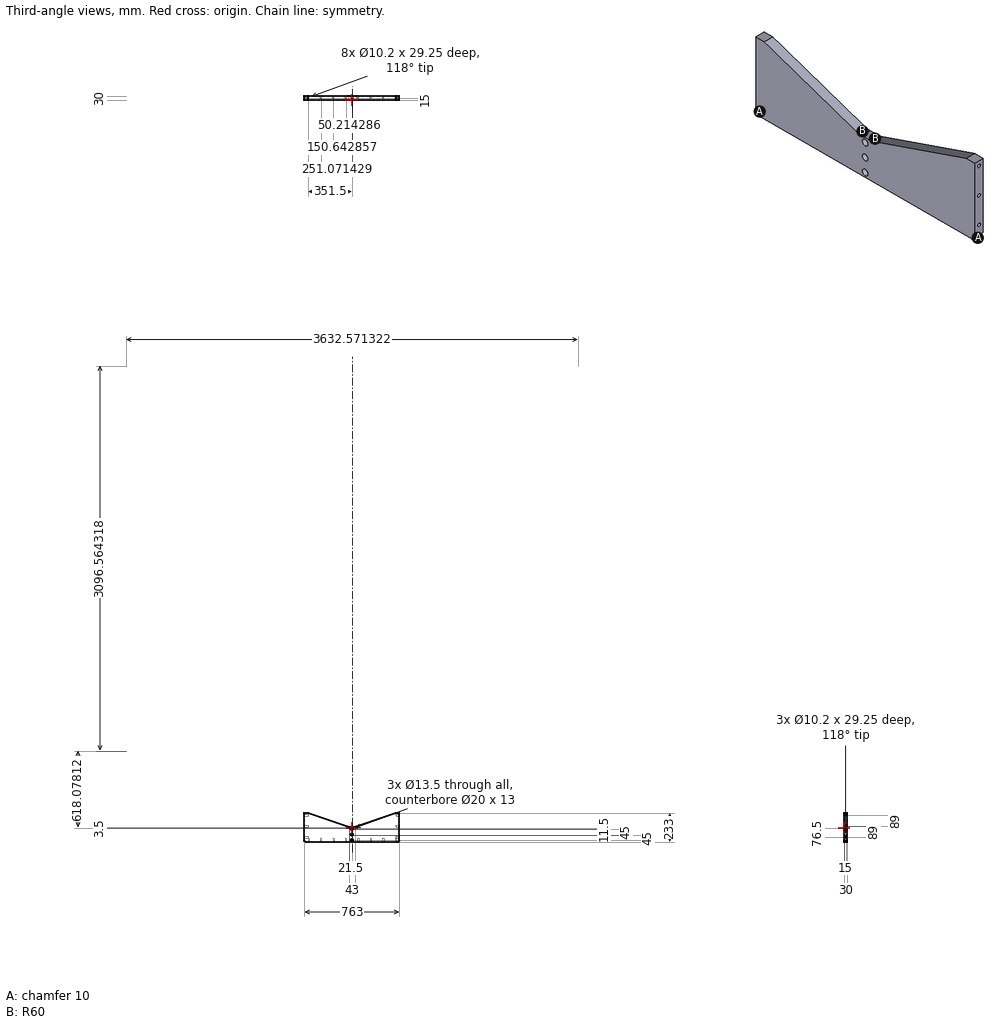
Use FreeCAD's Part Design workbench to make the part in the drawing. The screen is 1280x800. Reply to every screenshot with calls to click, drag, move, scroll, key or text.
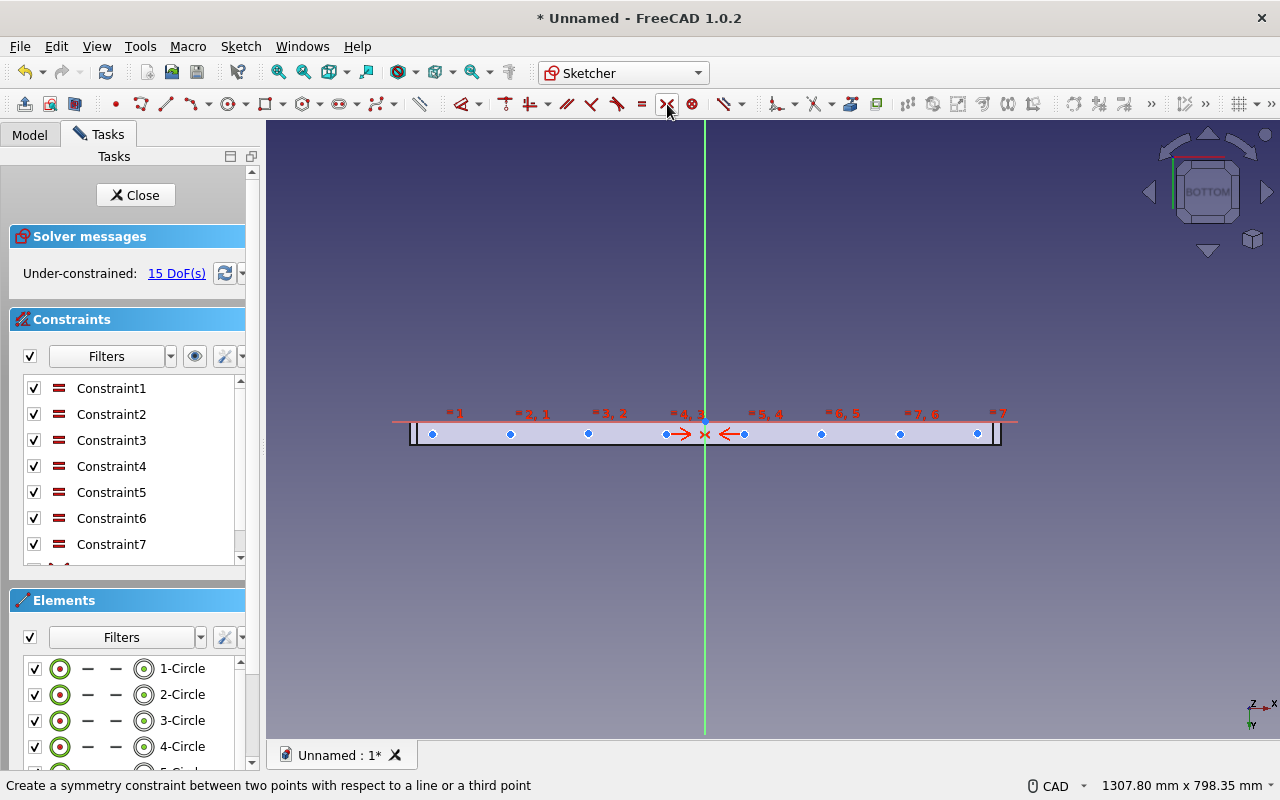
click(588, 434)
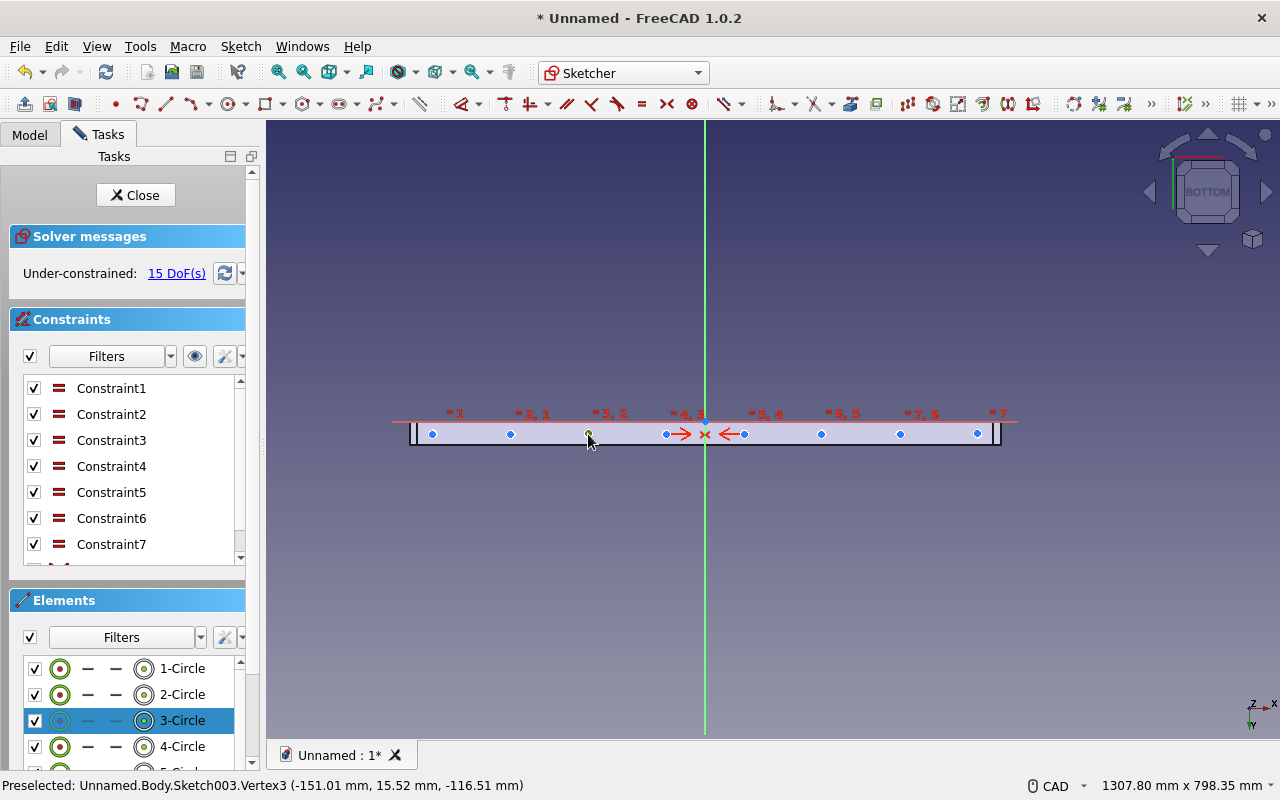
click(822, 434)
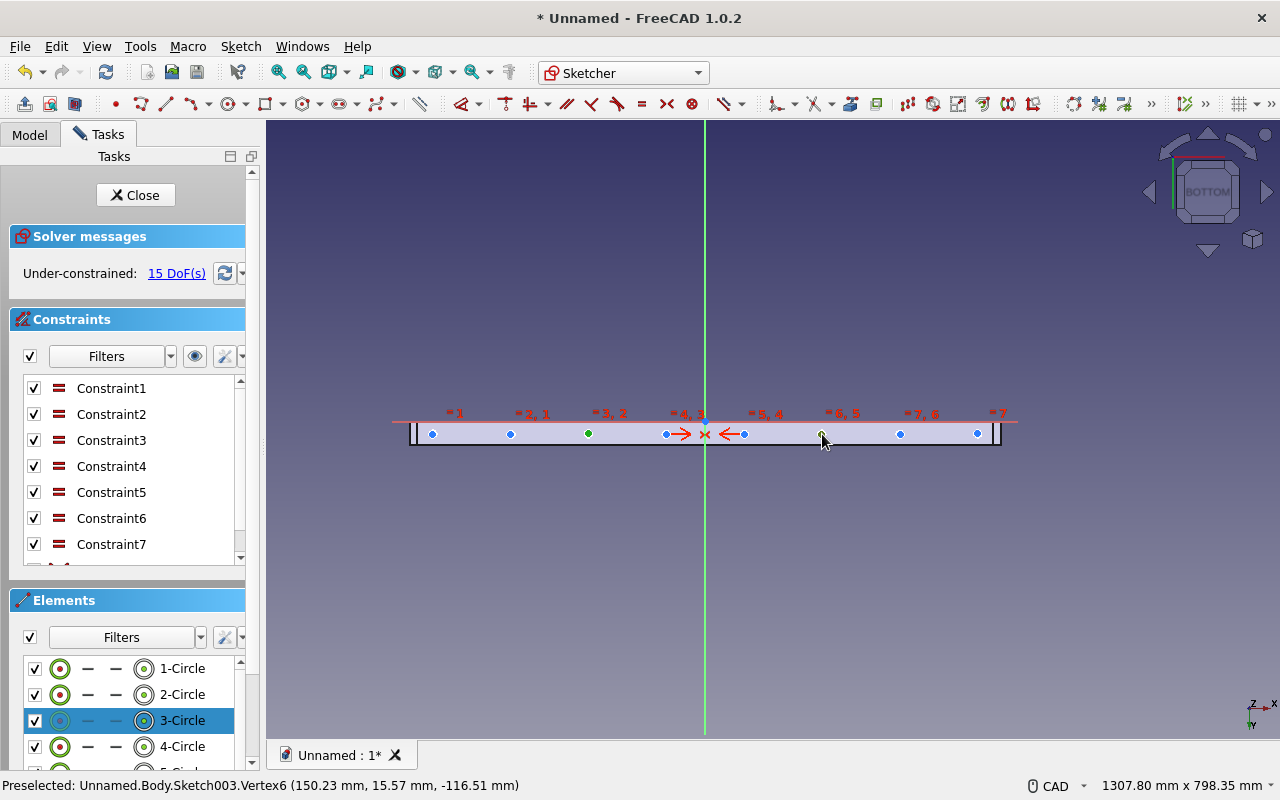
click(705, 671)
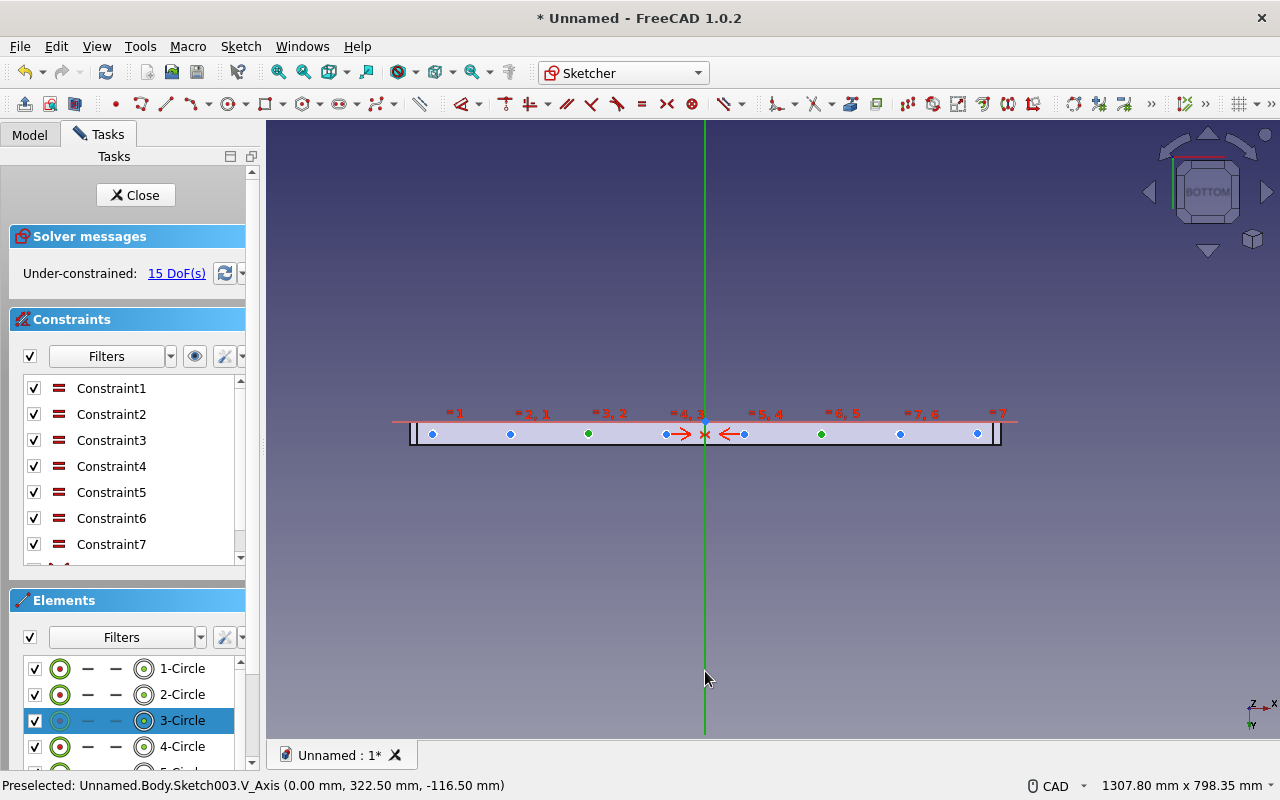
key(s)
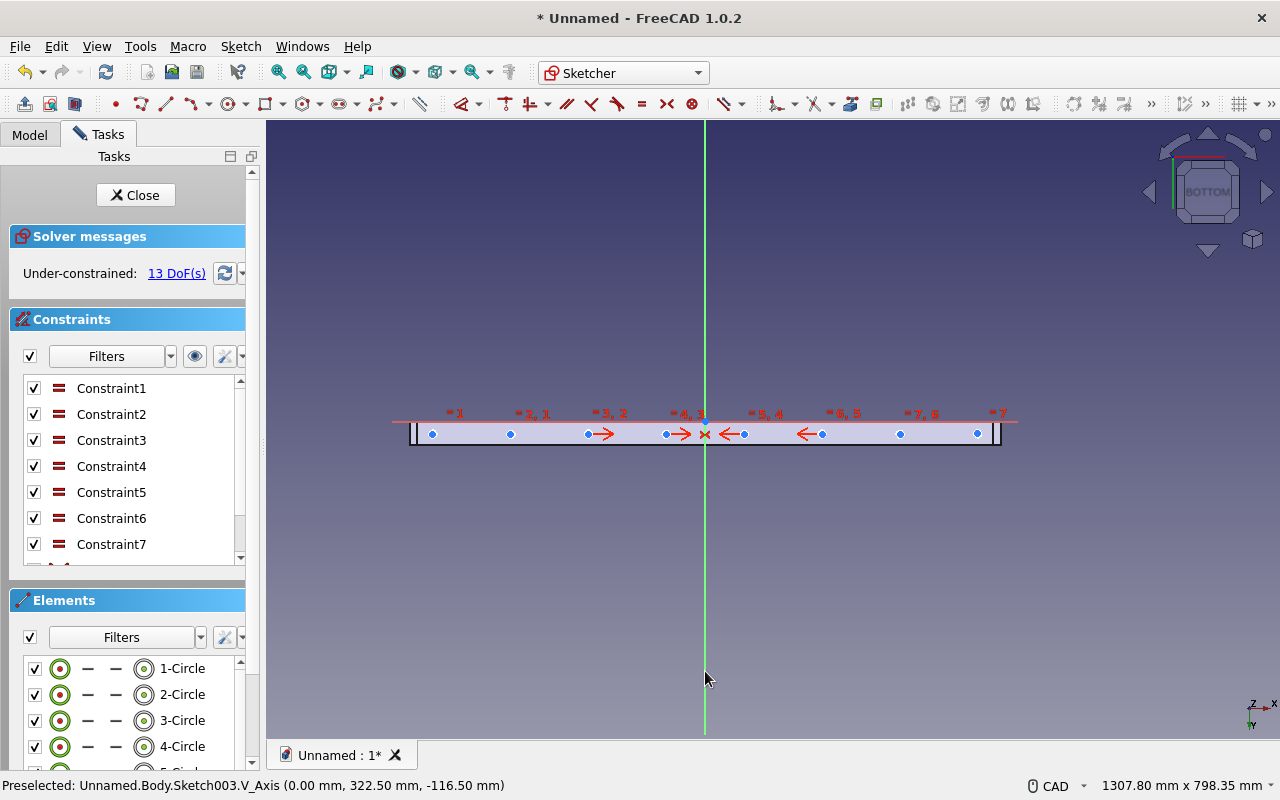
click(511, 435)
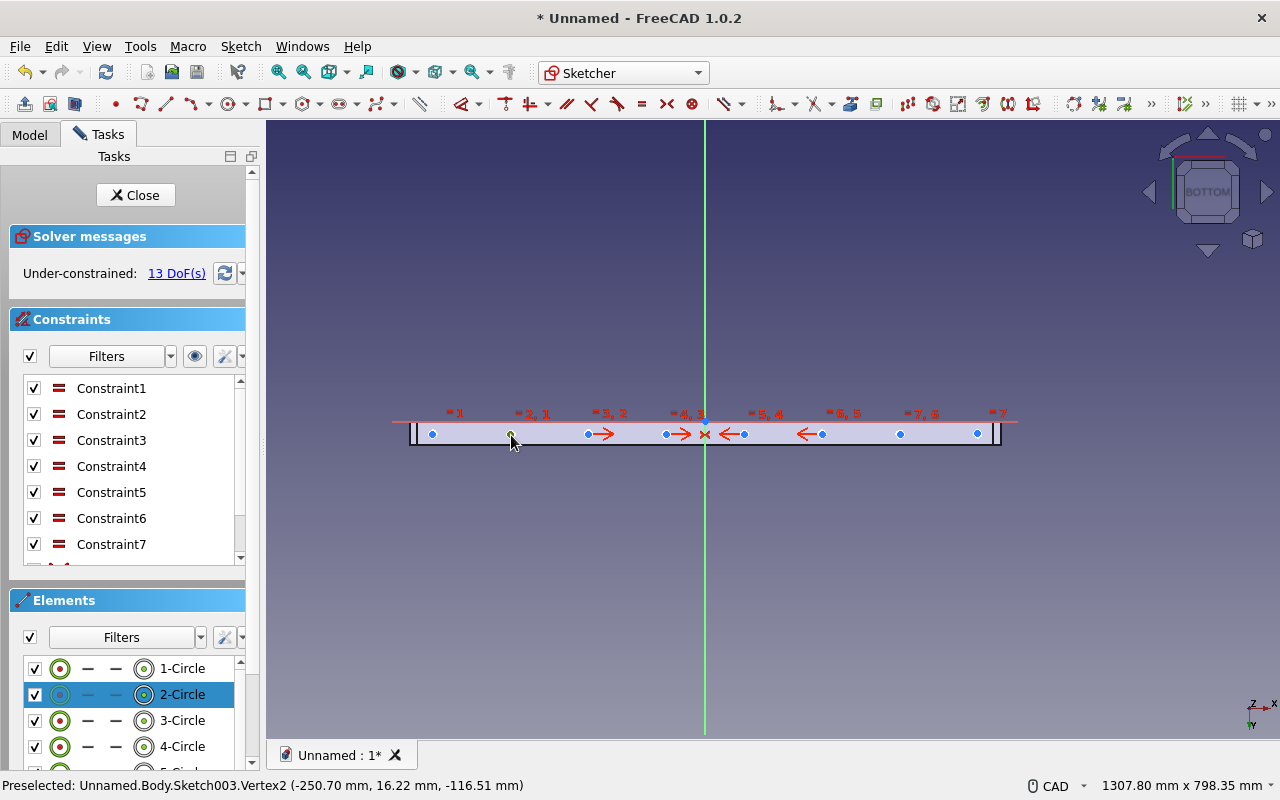
click(900, 434)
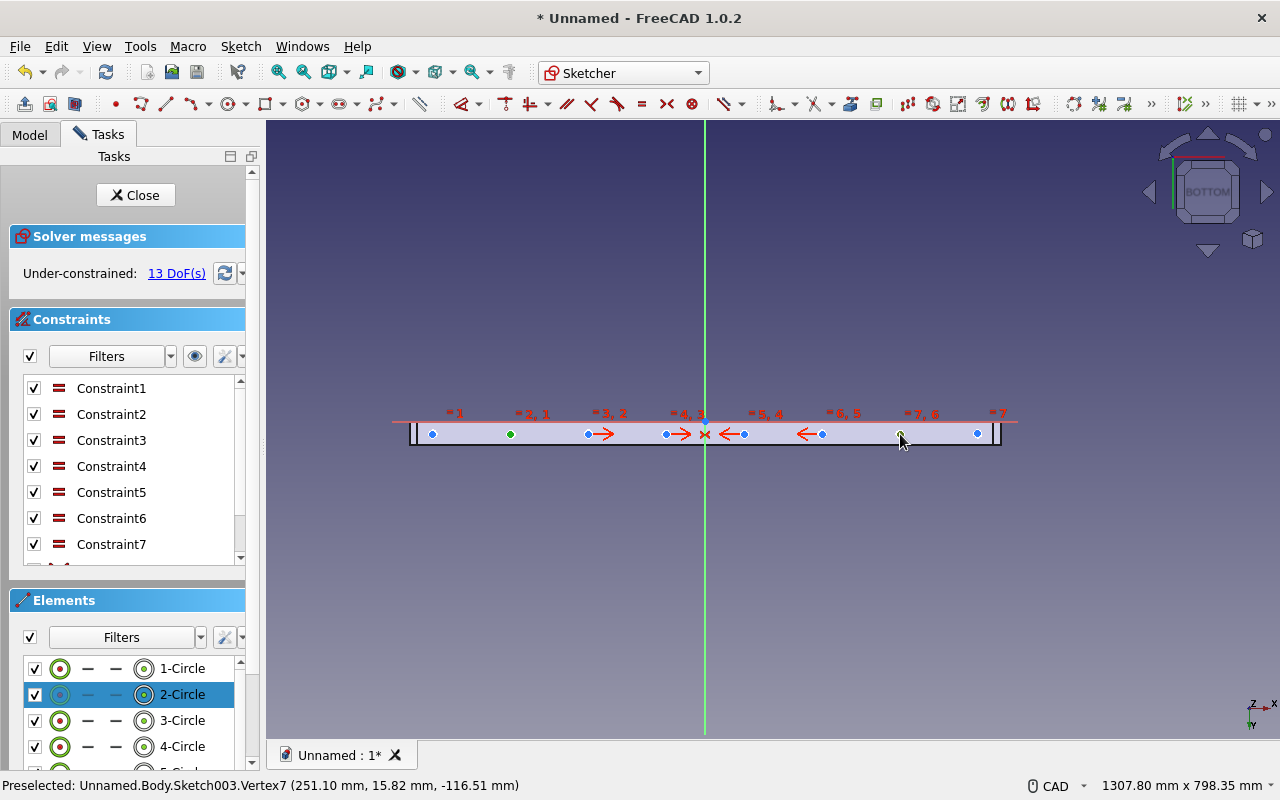
click(705, 671)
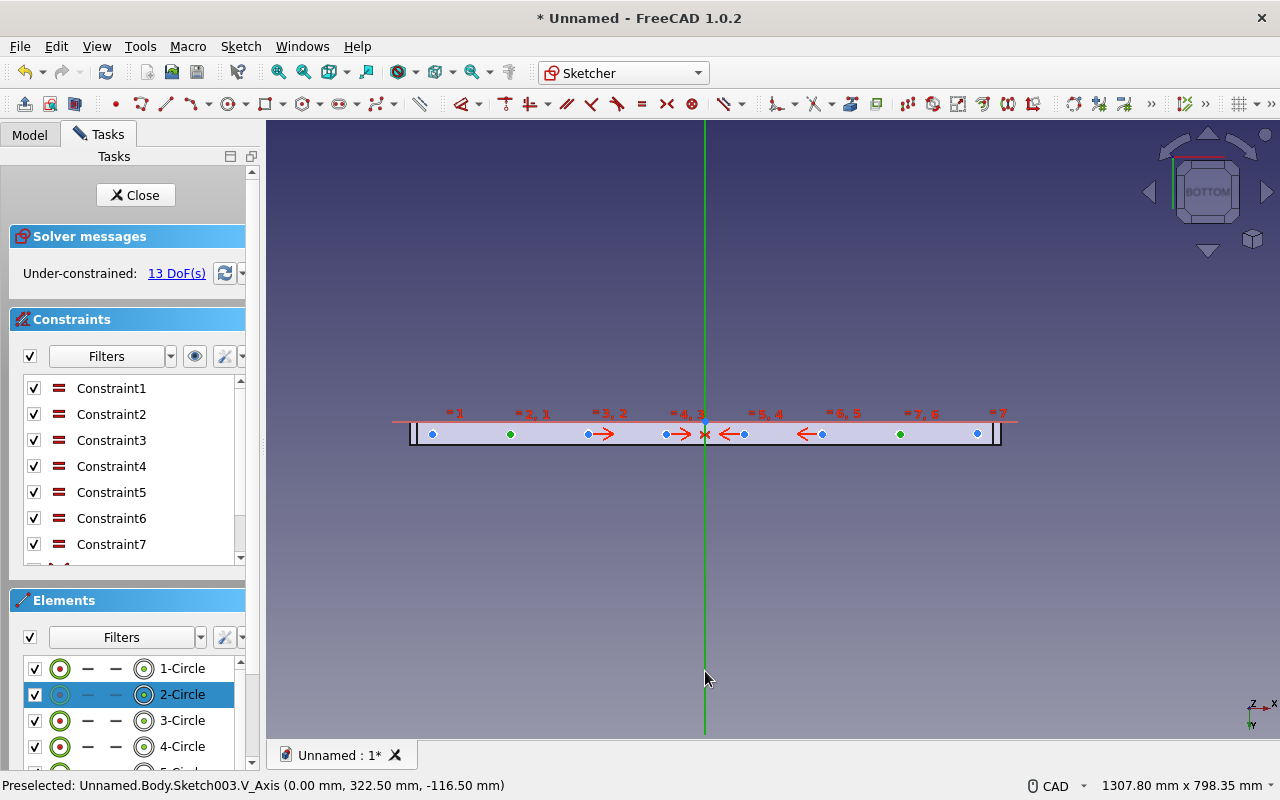
key(s)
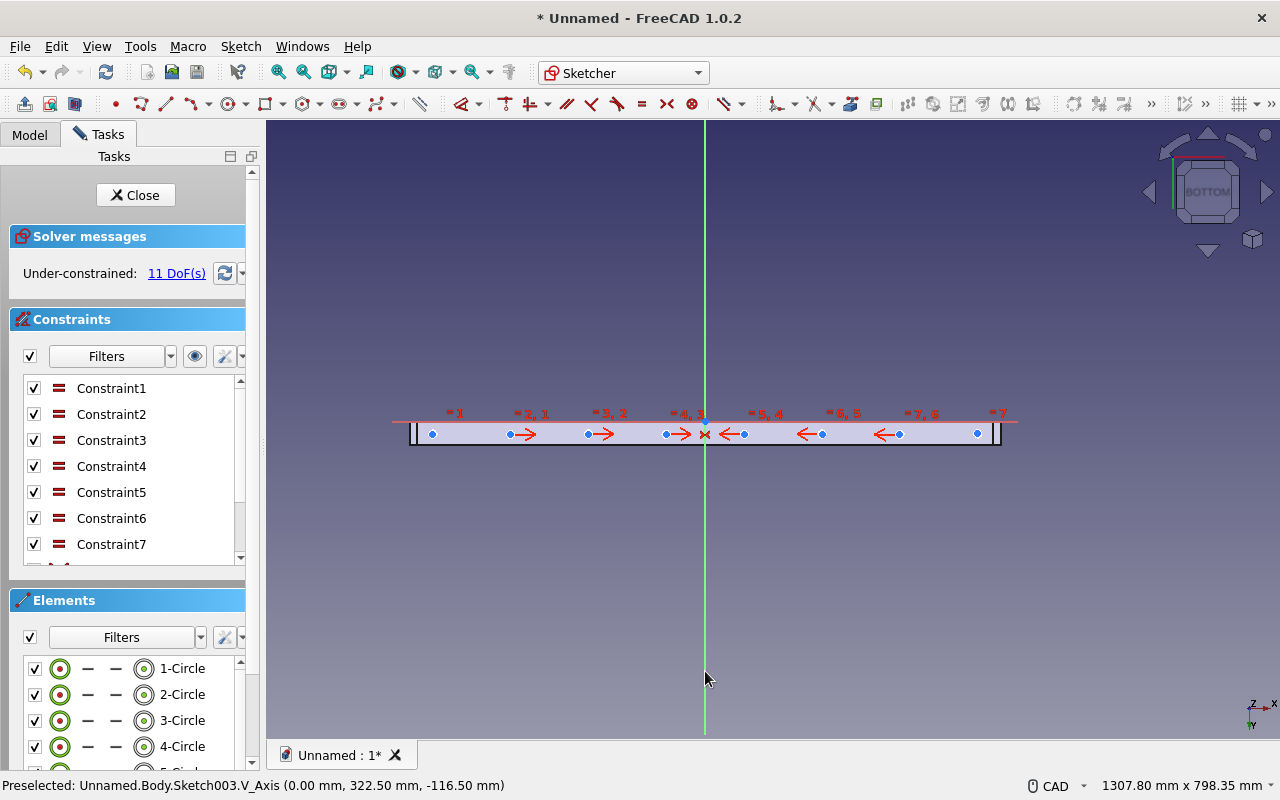
click(433, 434)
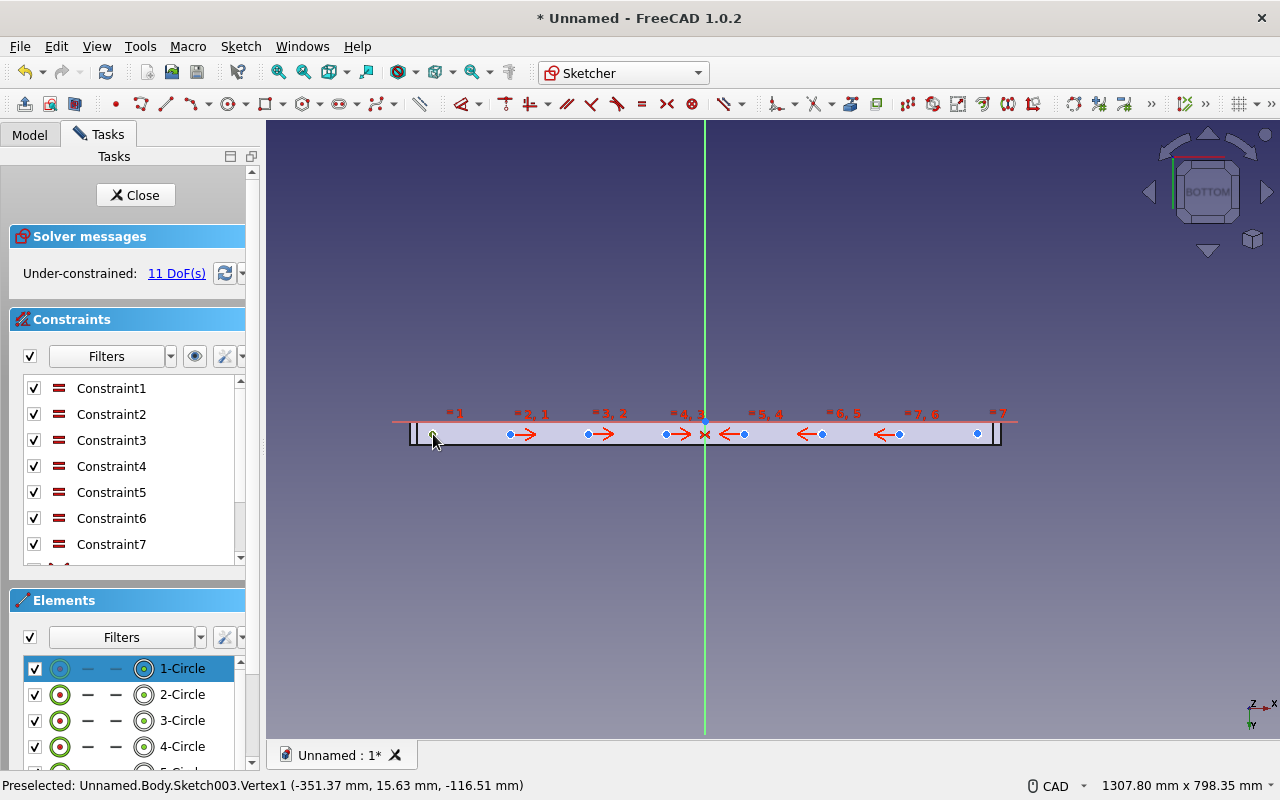
click(978, 434)